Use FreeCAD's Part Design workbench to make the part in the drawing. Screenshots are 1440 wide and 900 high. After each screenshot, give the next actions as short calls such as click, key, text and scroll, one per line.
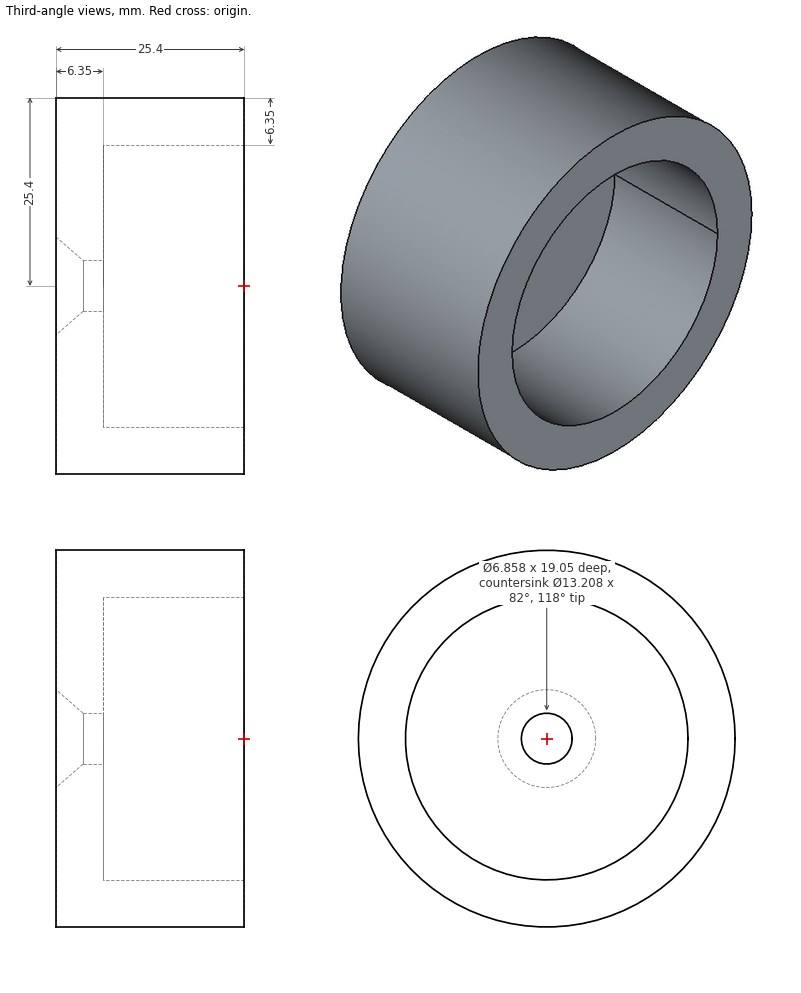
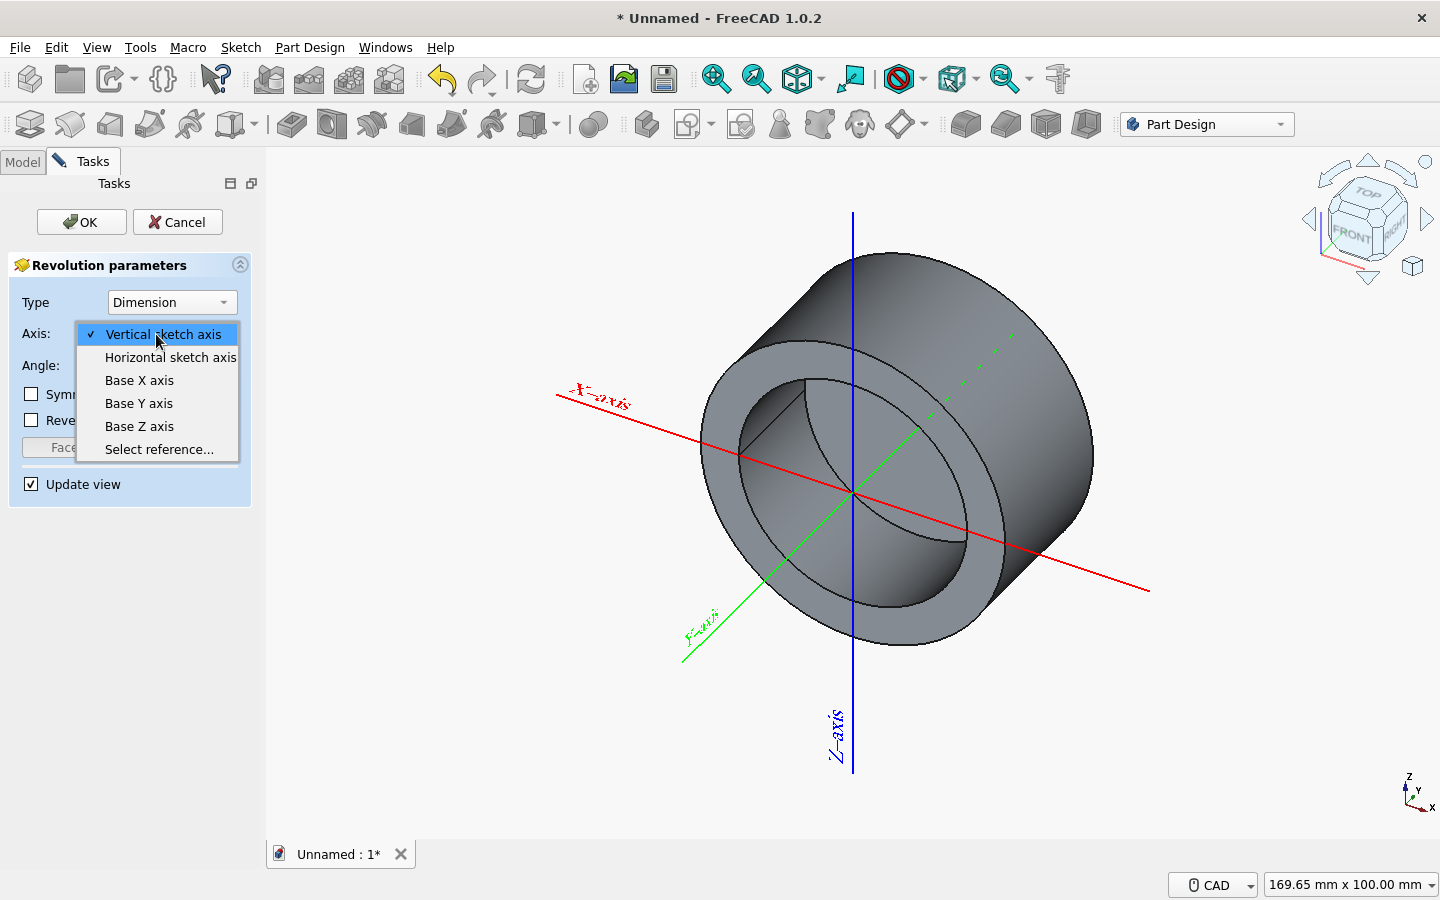
click(156, 358)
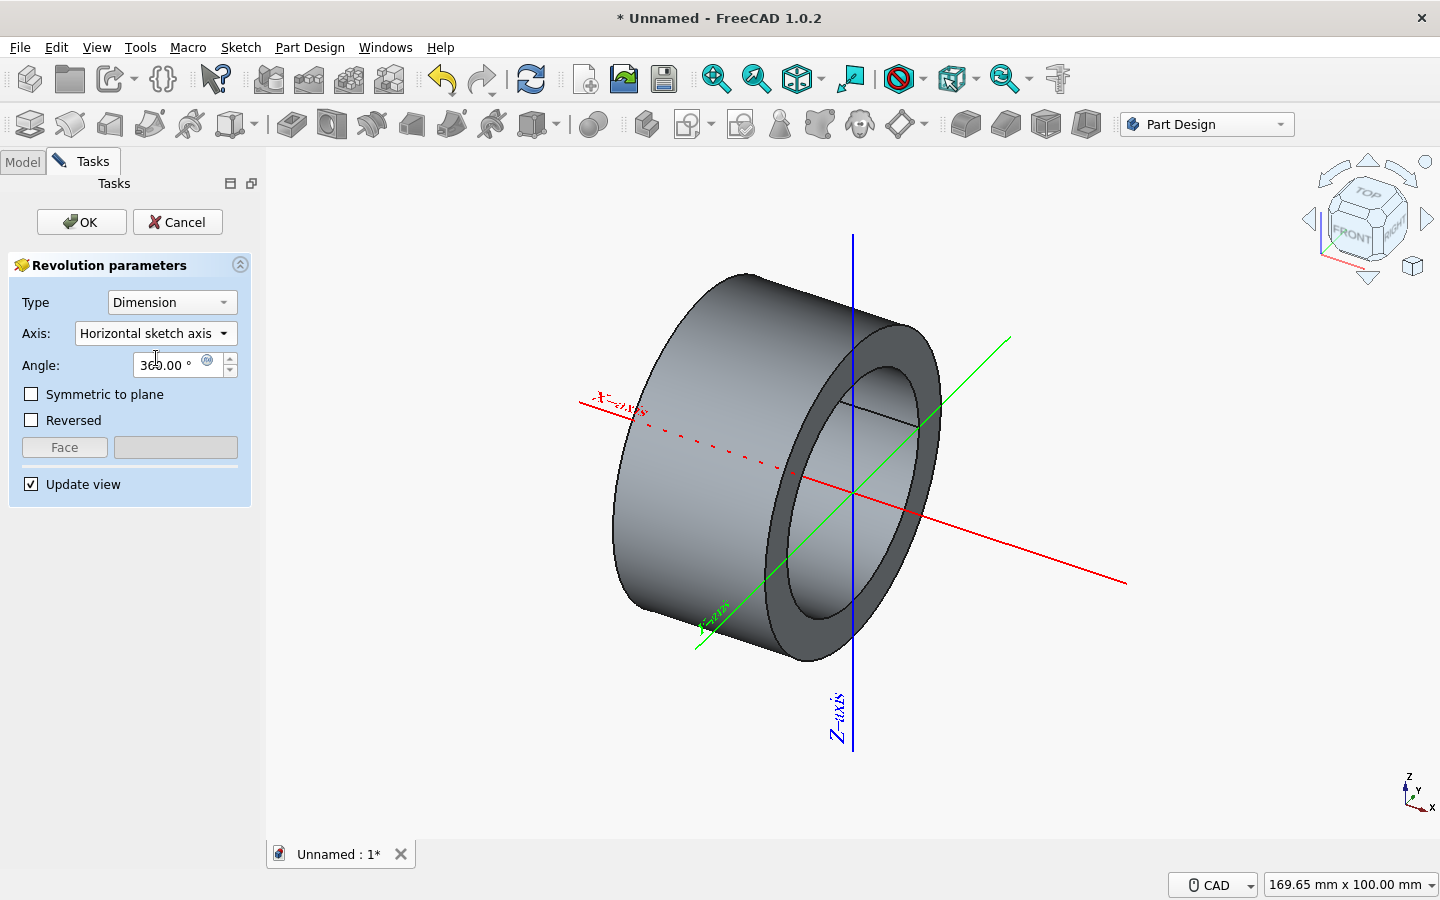
click(82, 222)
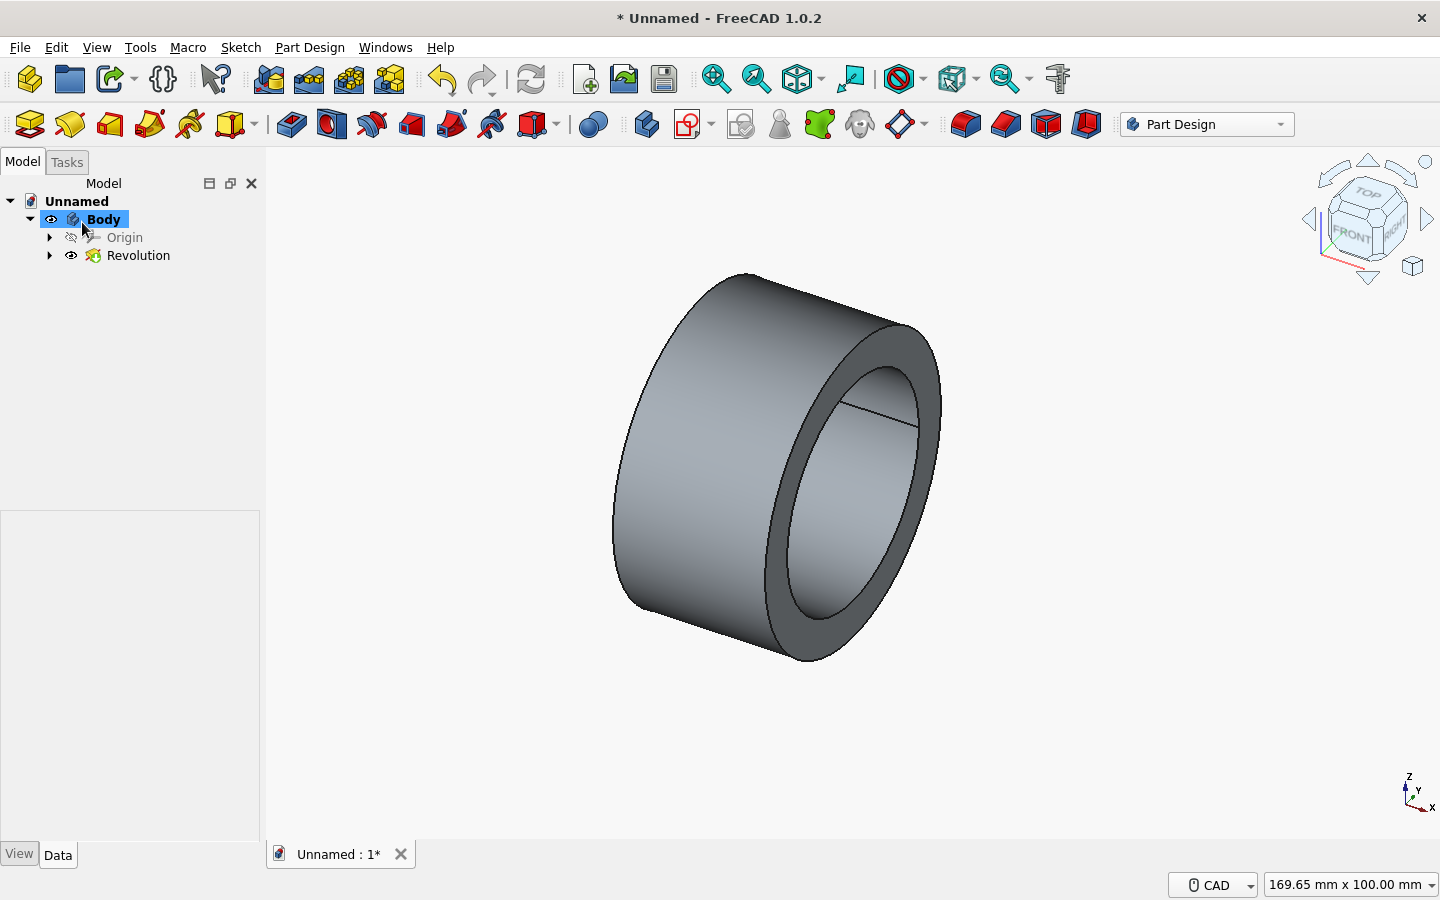
key(6)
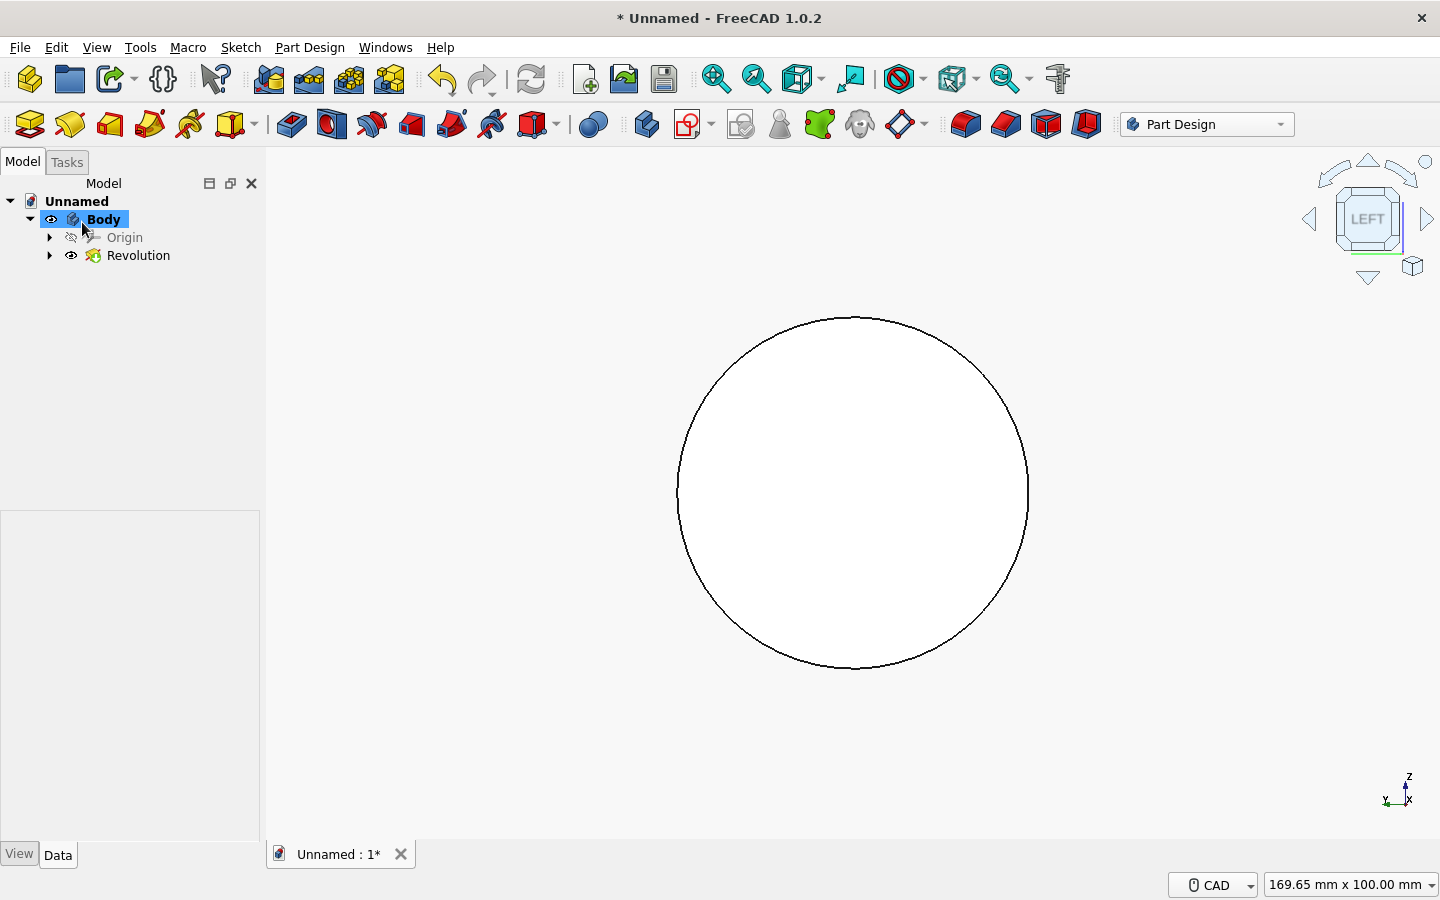
click(853, 492)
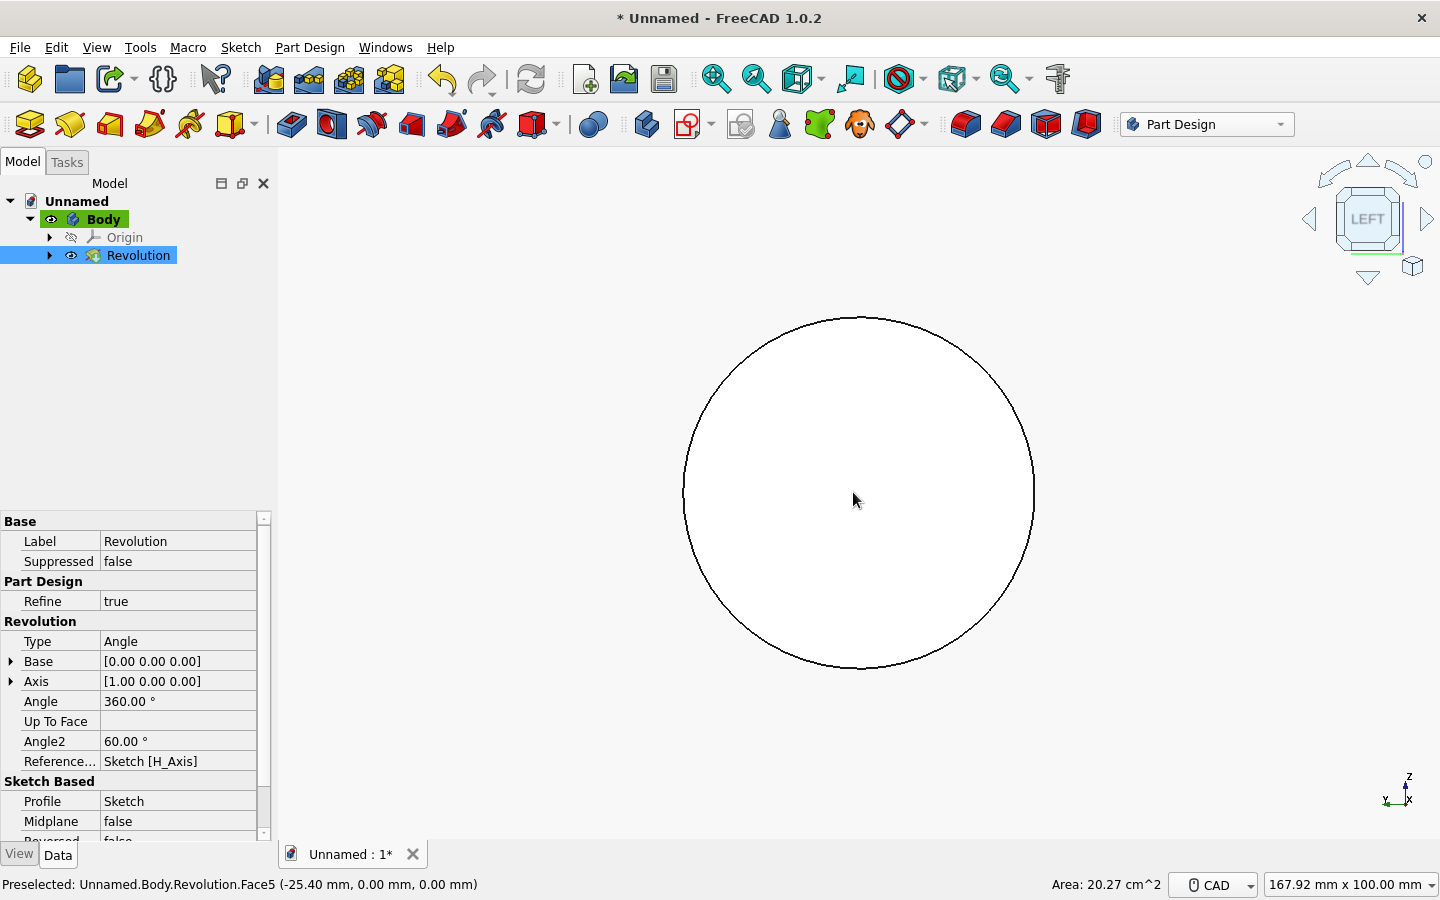
click(688, 124)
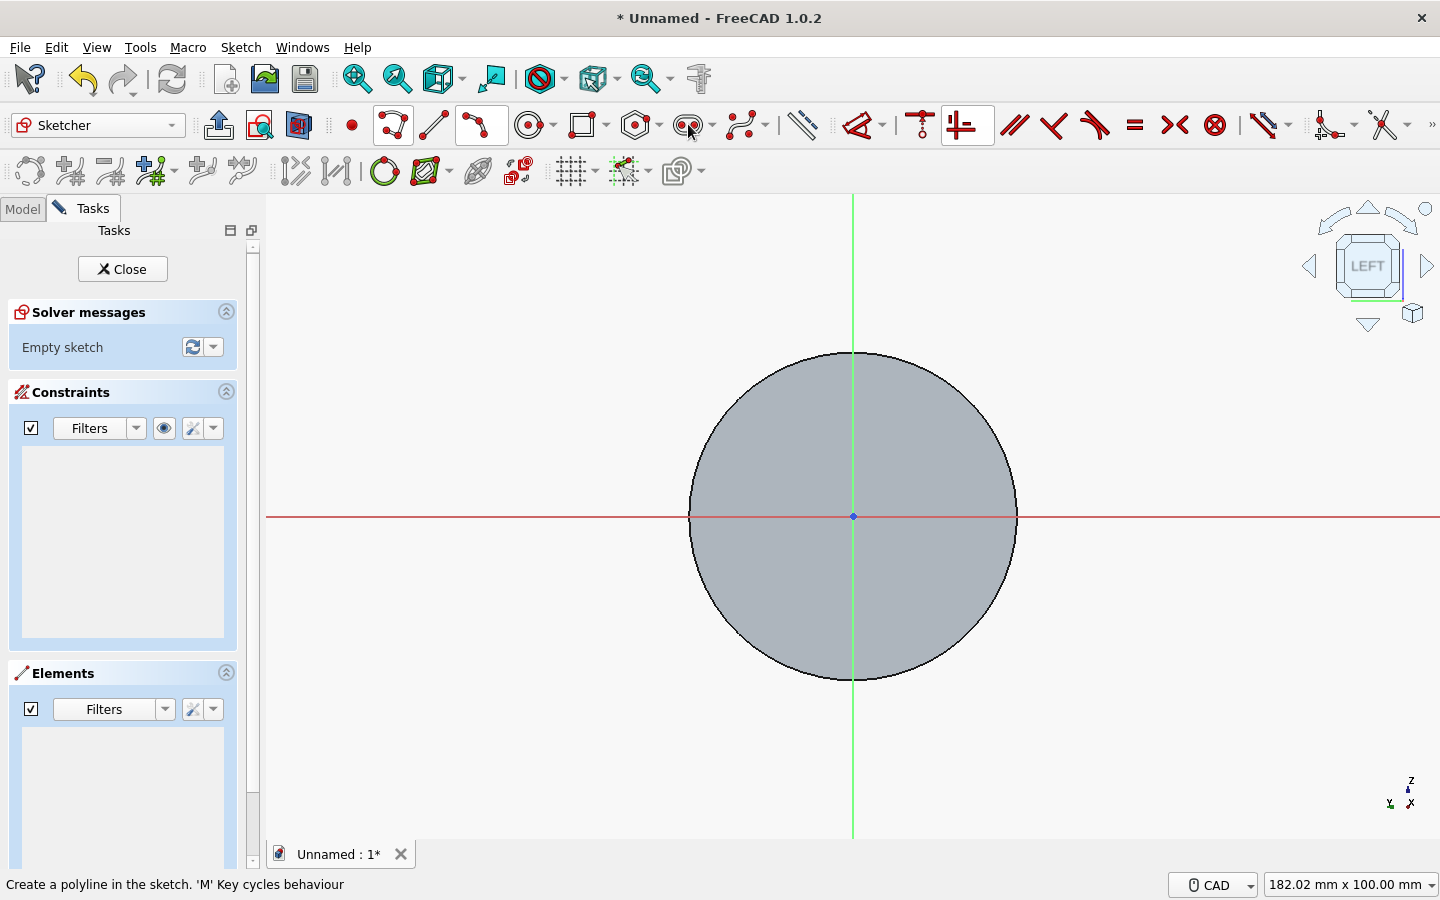
scroll(862, 516, up, 11)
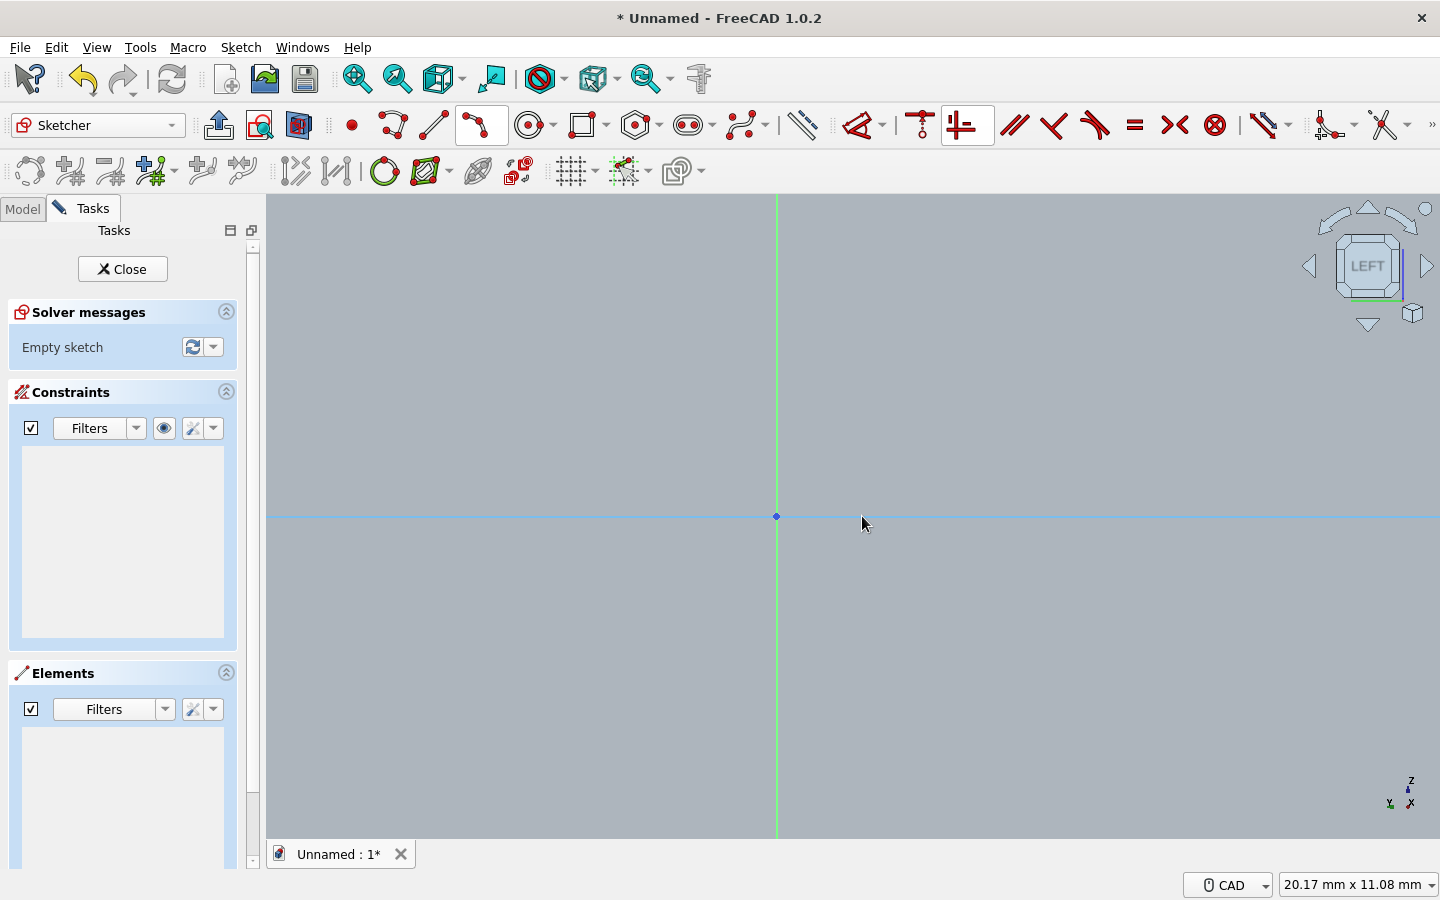
click(530, 126)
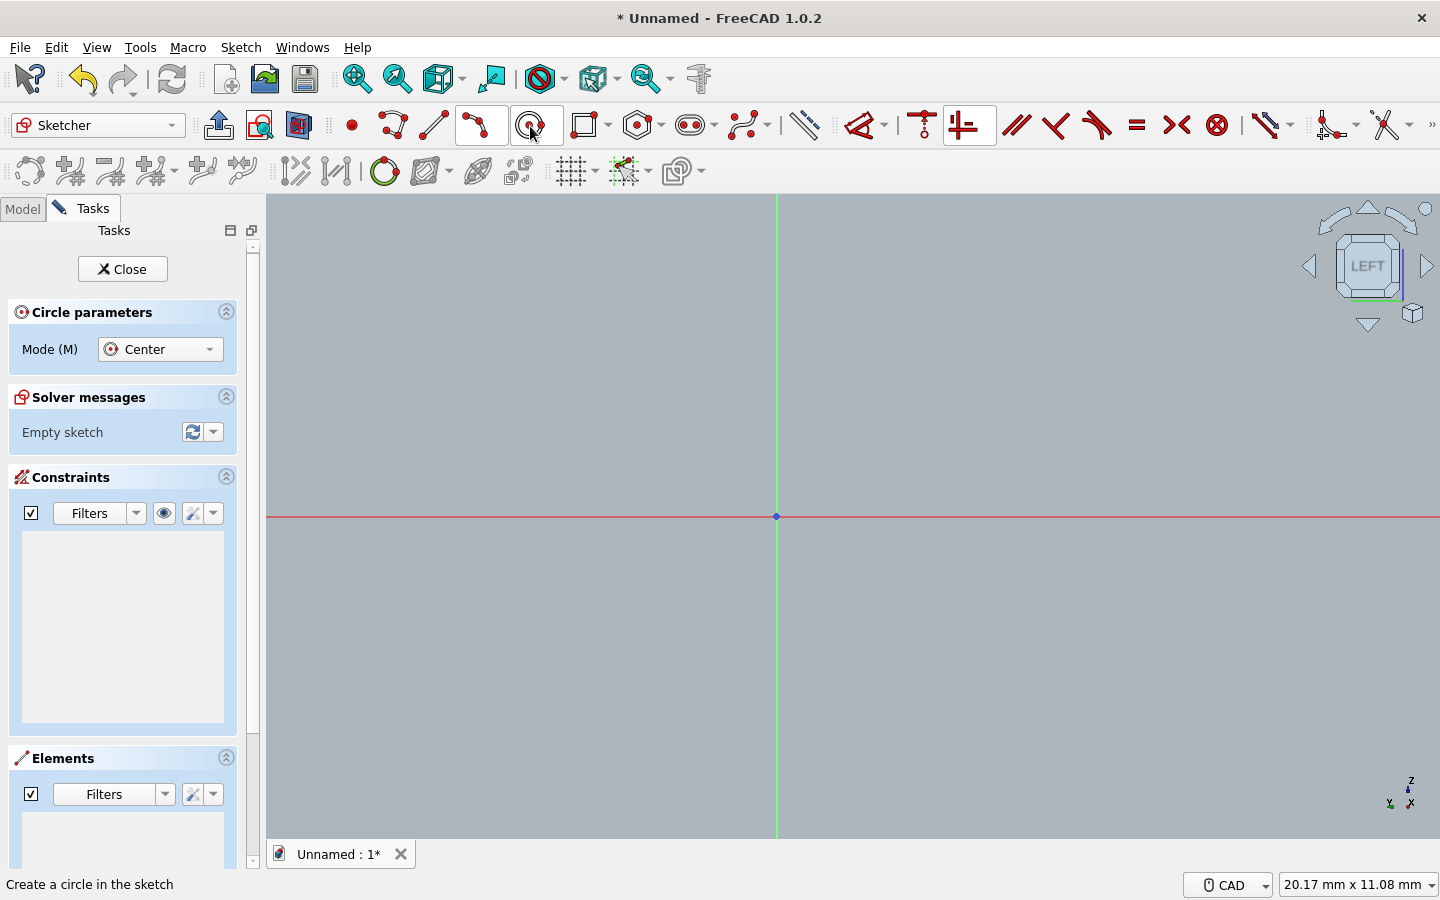
click(777, 516)
click(918, 375)
key(Escape)